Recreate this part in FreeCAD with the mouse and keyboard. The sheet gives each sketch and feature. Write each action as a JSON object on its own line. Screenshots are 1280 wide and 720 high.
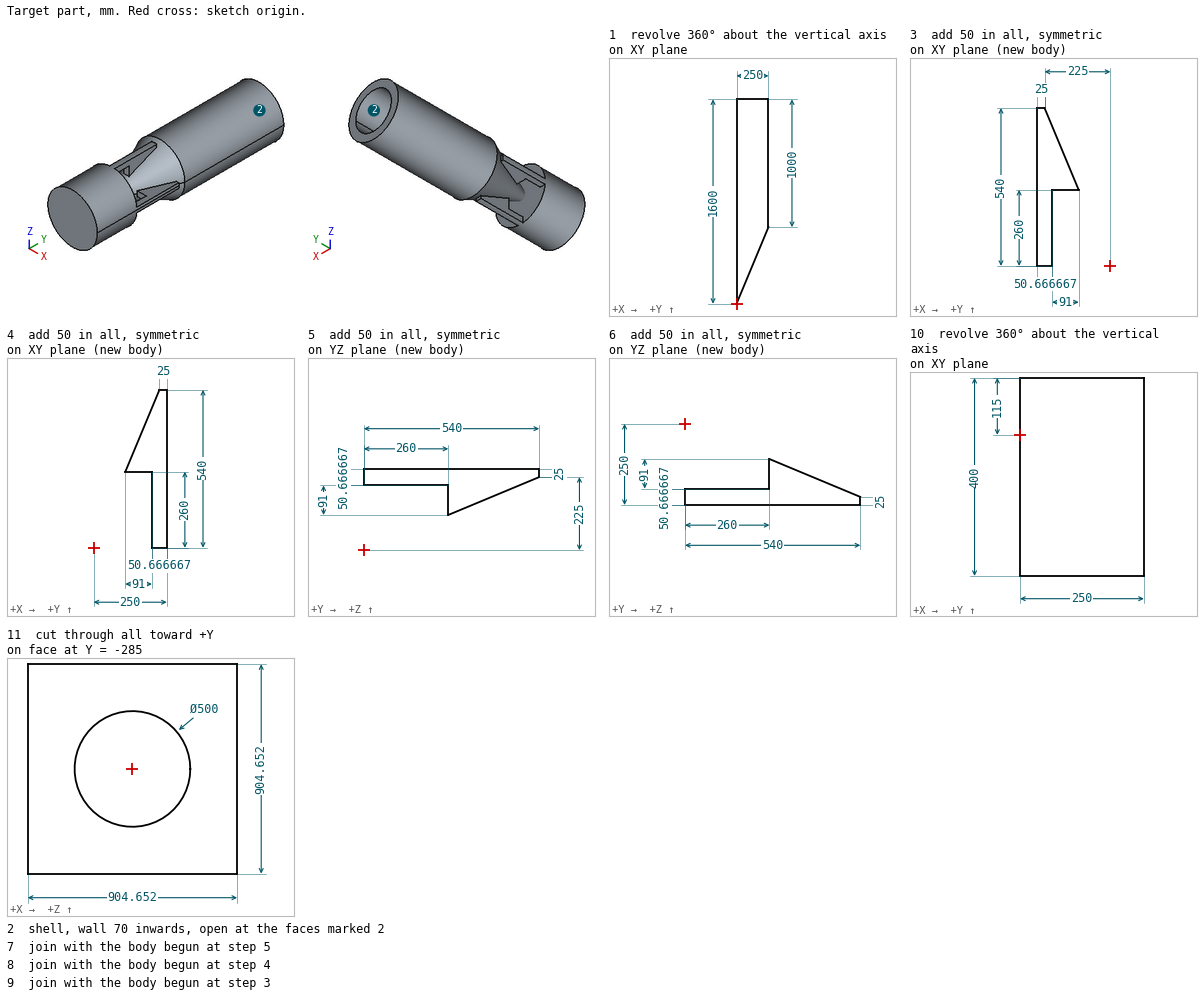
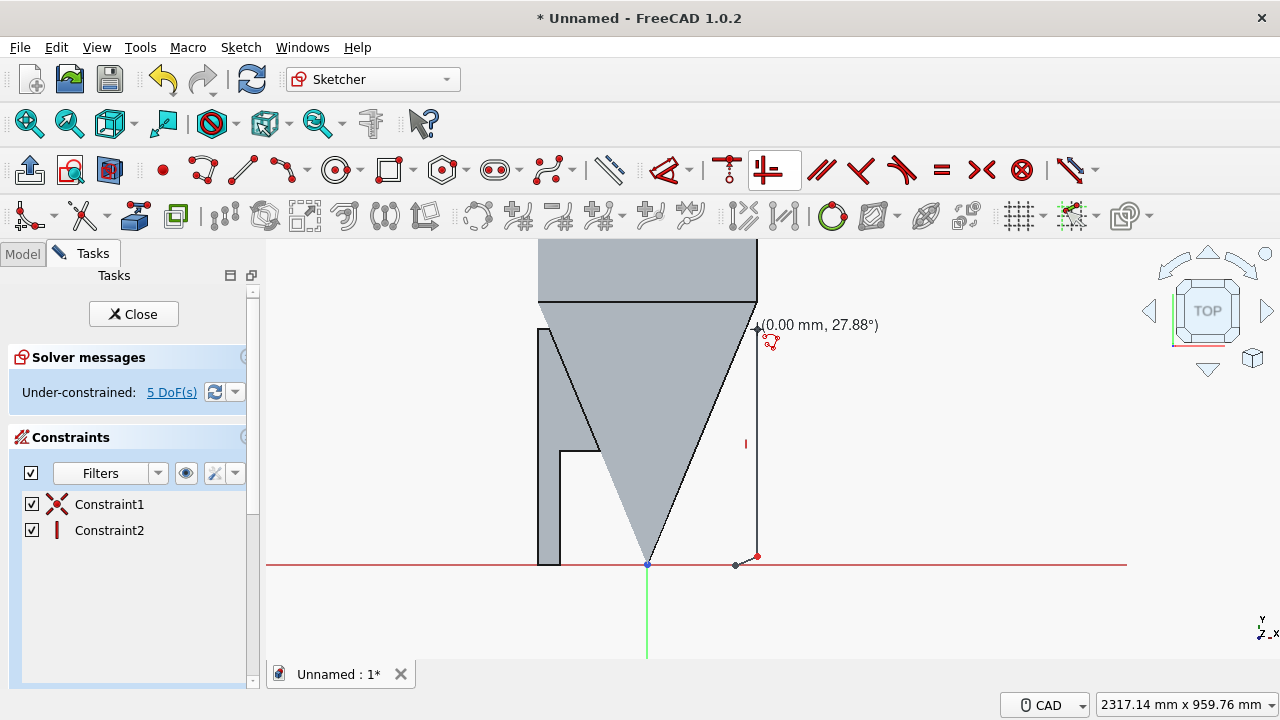
{"action": "scroll", "coordinate": [746, 329], "scroll_direction": "up", "scroll_amount": 2}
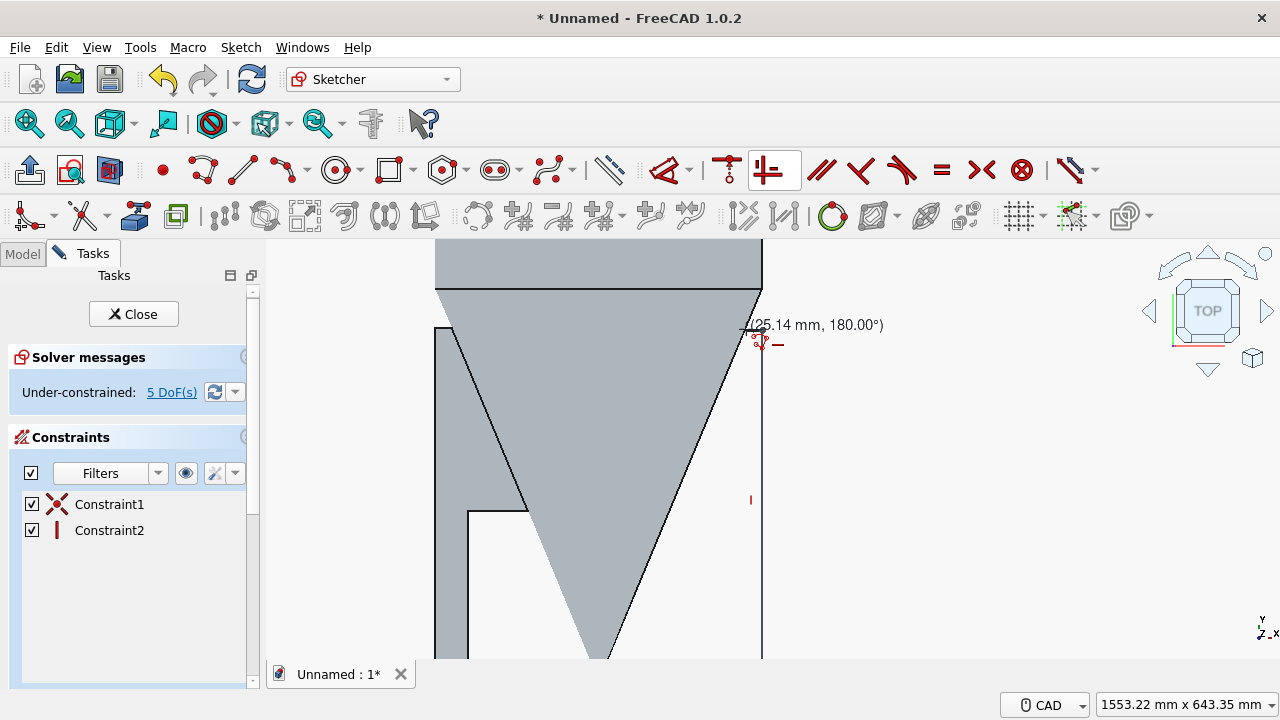
{"action": "left_click", "coordinate": [745, 329]}
{"action": "left_click", "coordinate": [669, 511]}
{"action": "left_click", "coordinate": [729, 511]}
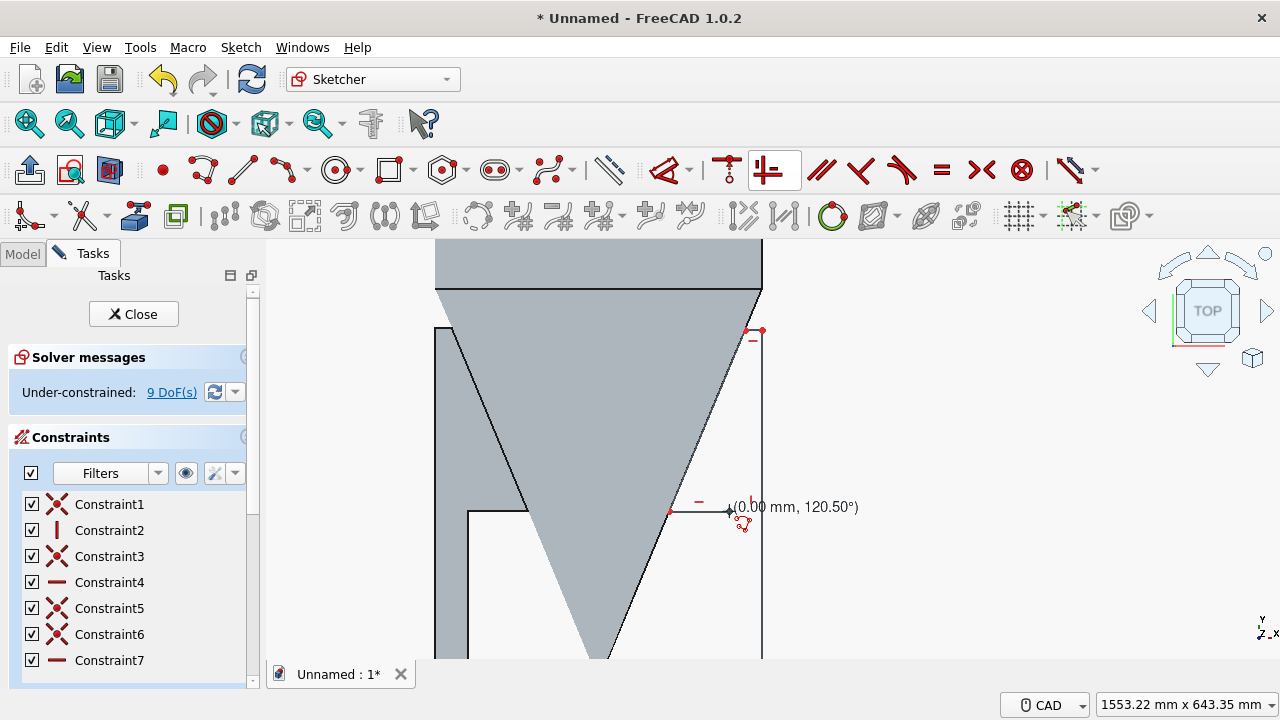
{"action": "scroll", "coordinate": [754, 336], "scroll_direction": "down", "scroll_amount": 2}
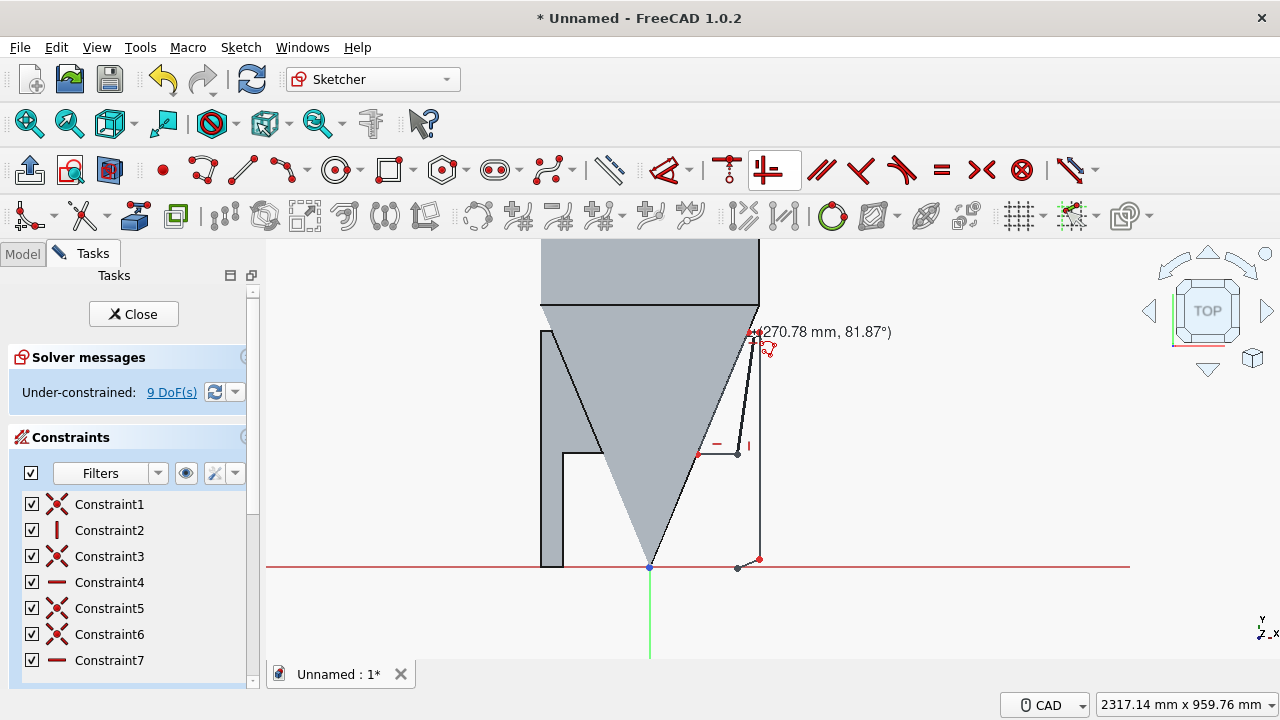
{"action": "scroll", "coordinate": [737, 567], "scroll_direction": "up", "scroll_amount": 2}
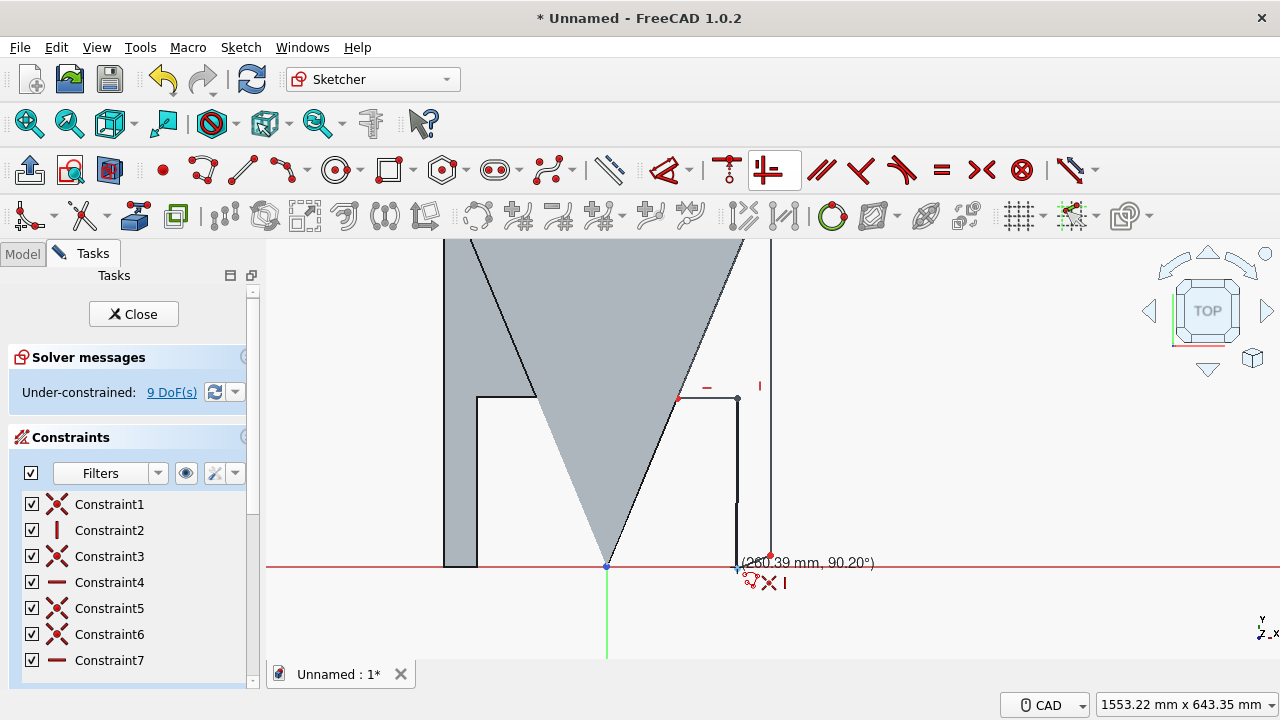
{"action": "left_click", "coordinate": [738, 569]}
{"action": "key", "text": "Escape"}
{"action": "key", "text": "Escape"}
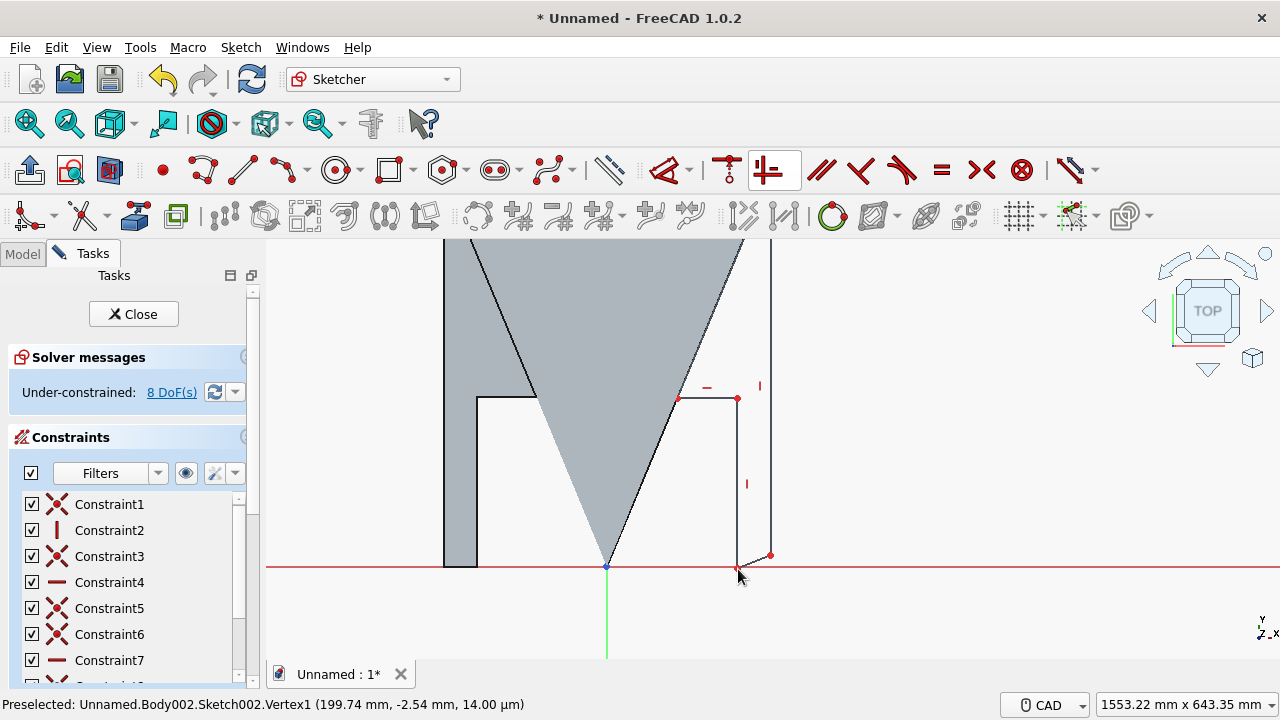
{"action": "scroll", "coordinate": [747, 565], "scroll_direction": "up", "scroll_amount": 2}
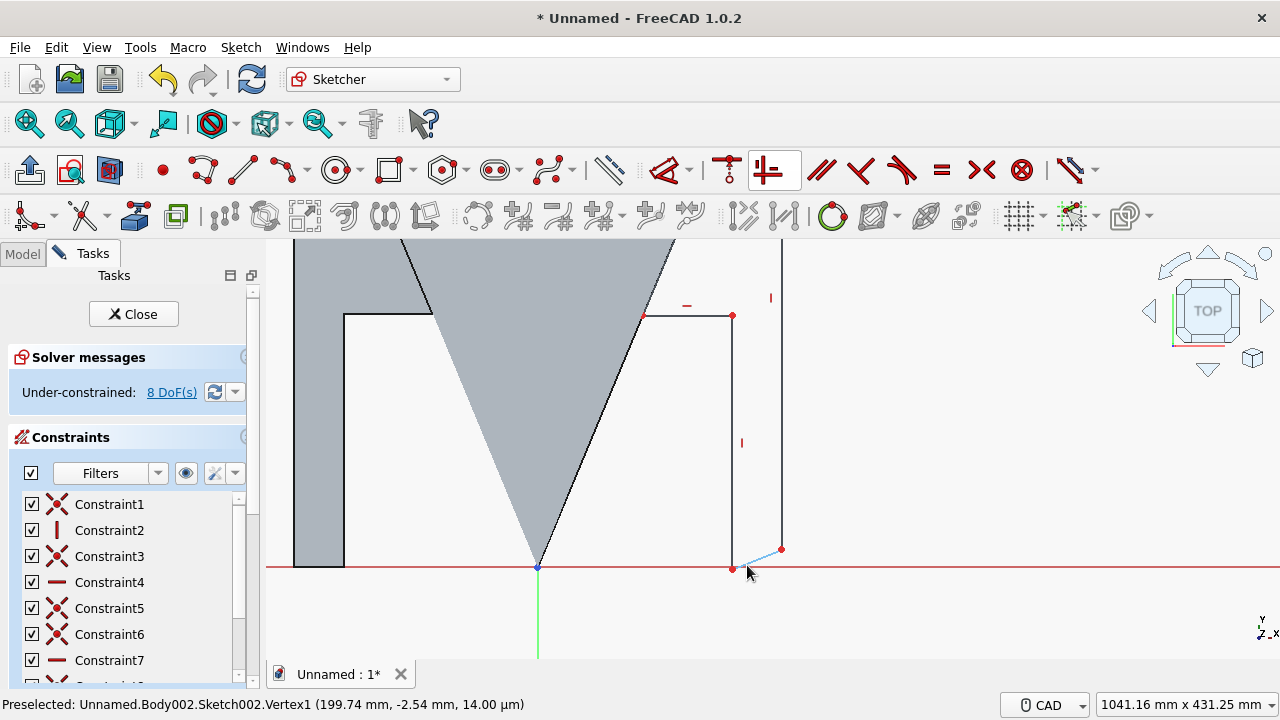
{"action": "left_click", "coordinate": [747, 564]}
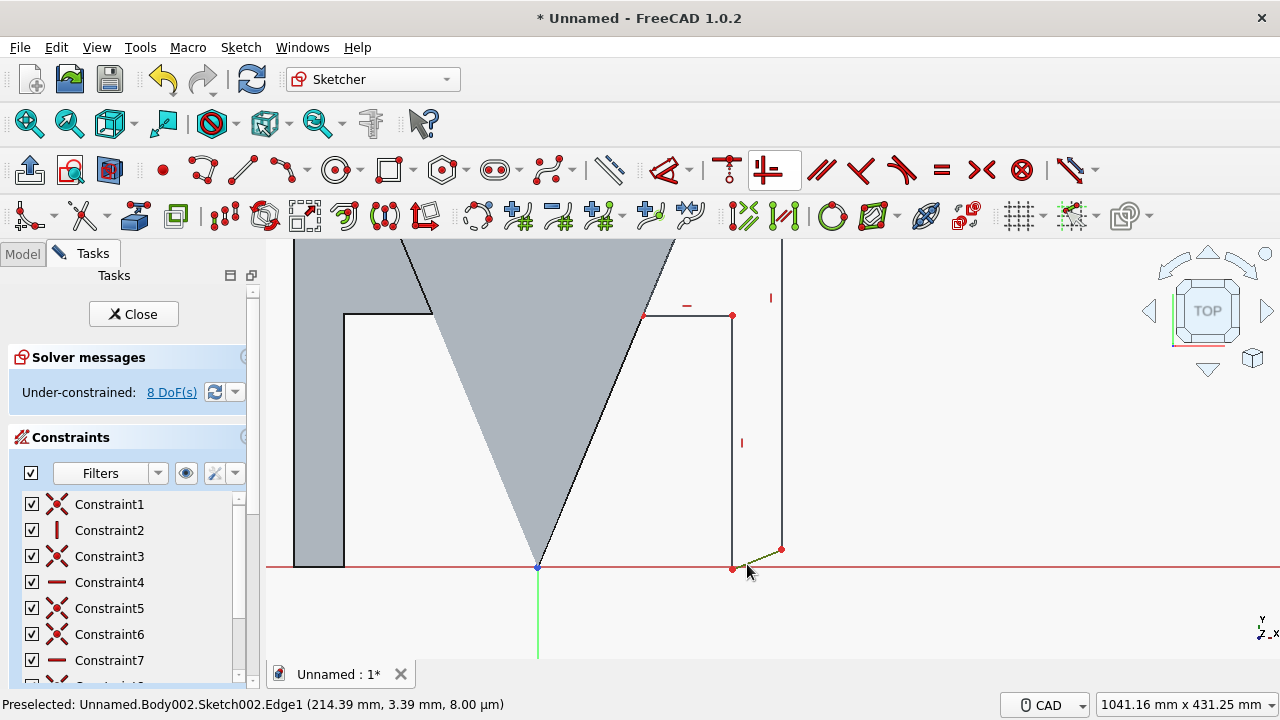
{"action": "left_click", "coordinate": [796, 170]}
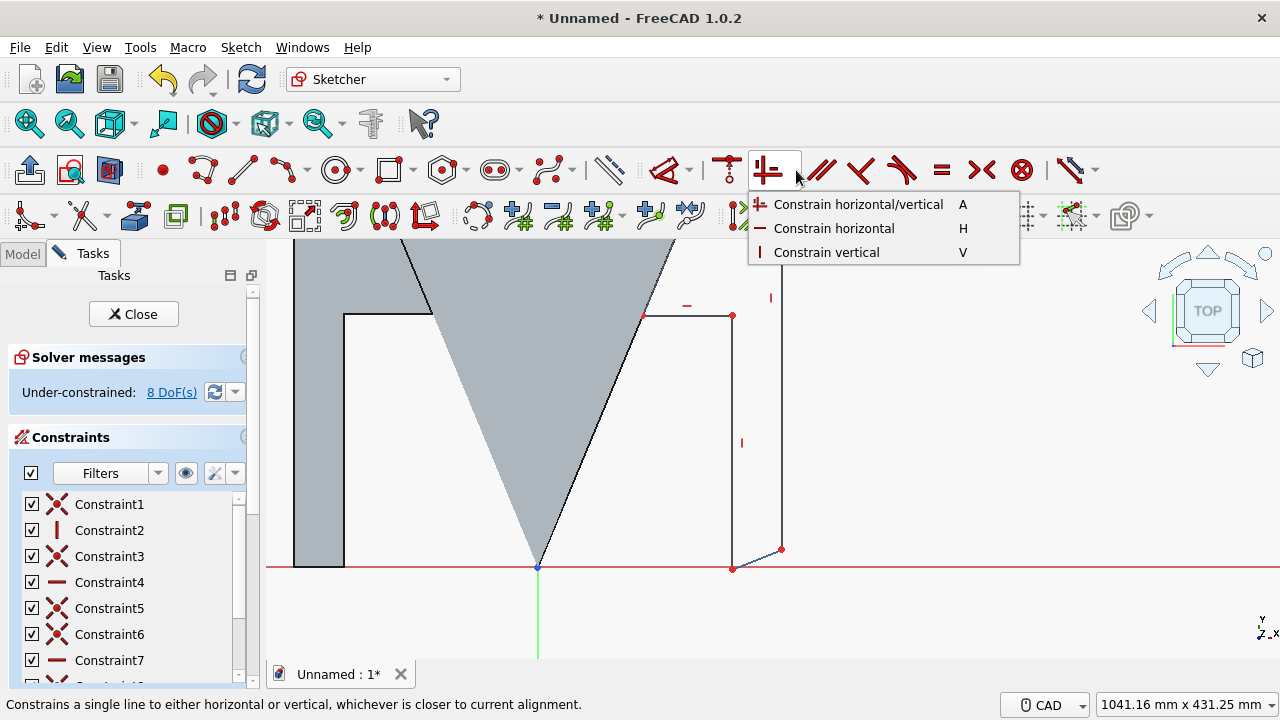
{"action": "left_click", "coordinate": [884, 228]}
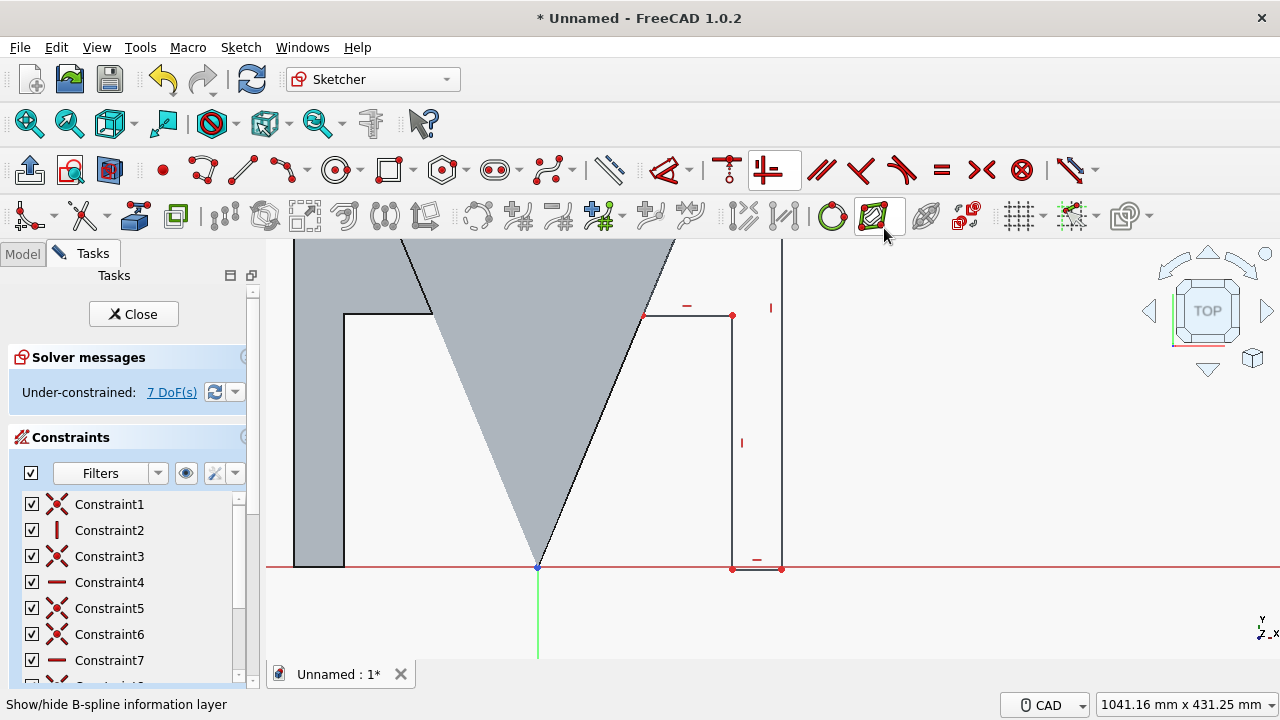
{"action": "left_click", "coordinate": [732, 570]}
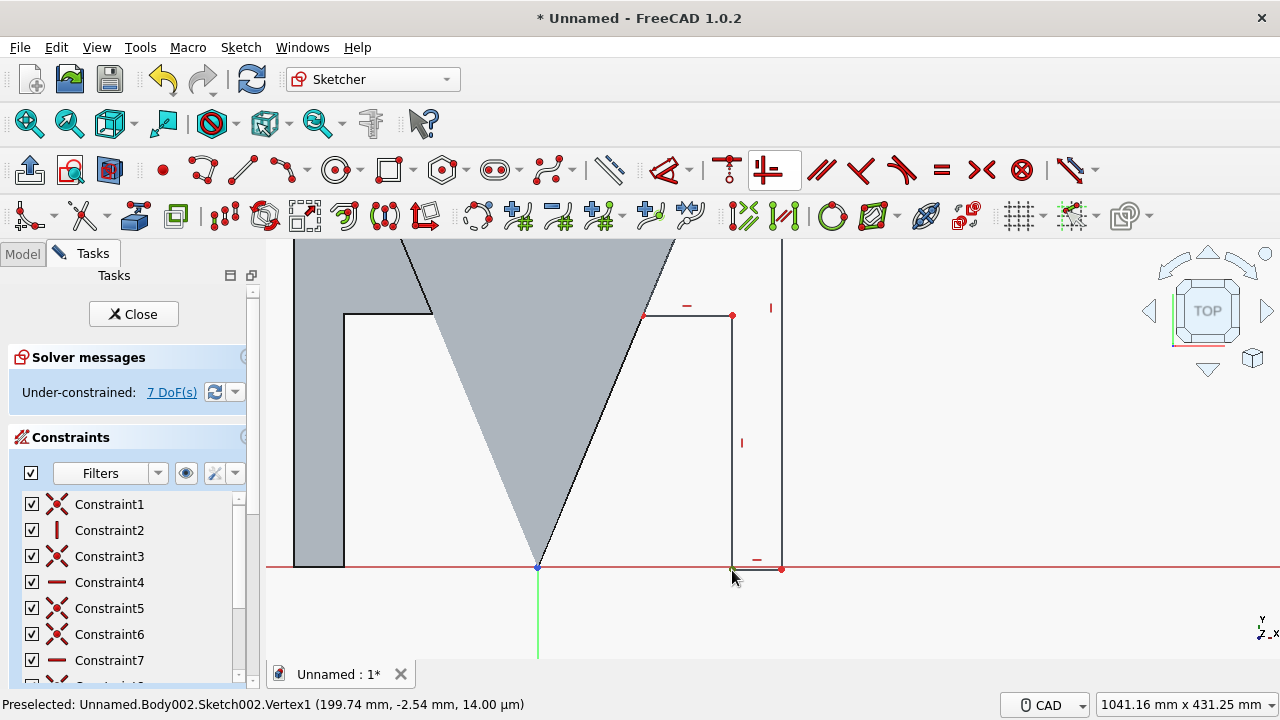
{"action": "left_click", "coordinate": [353, 567]}